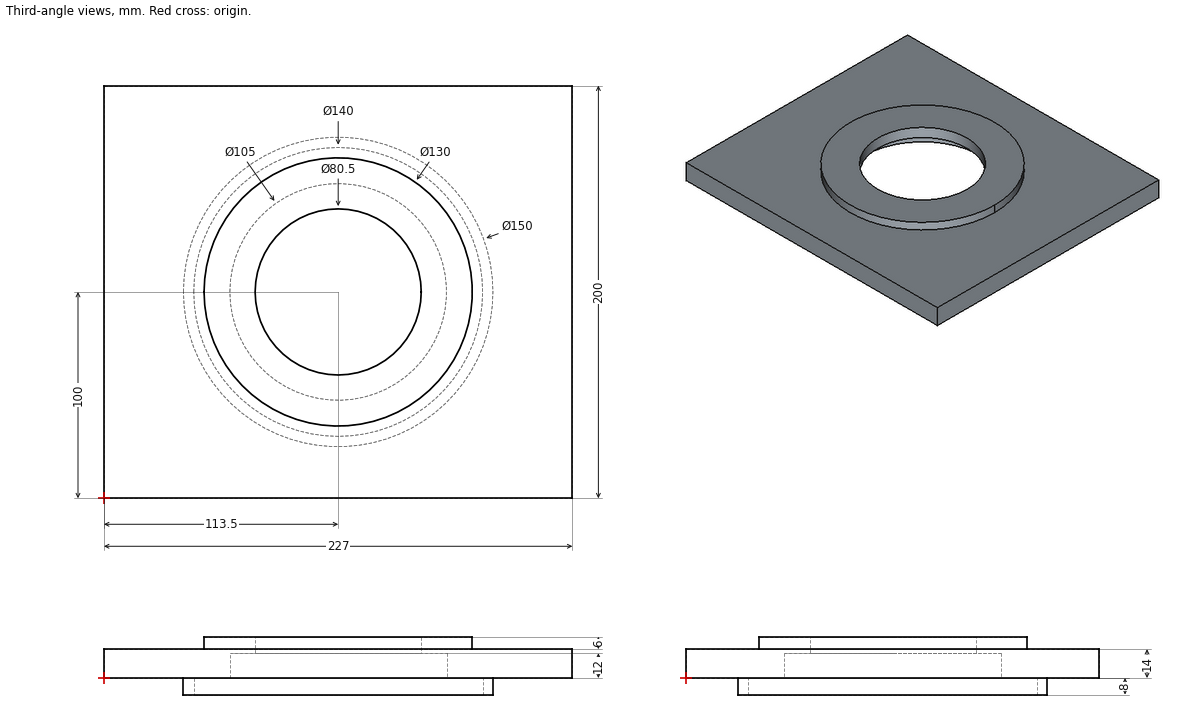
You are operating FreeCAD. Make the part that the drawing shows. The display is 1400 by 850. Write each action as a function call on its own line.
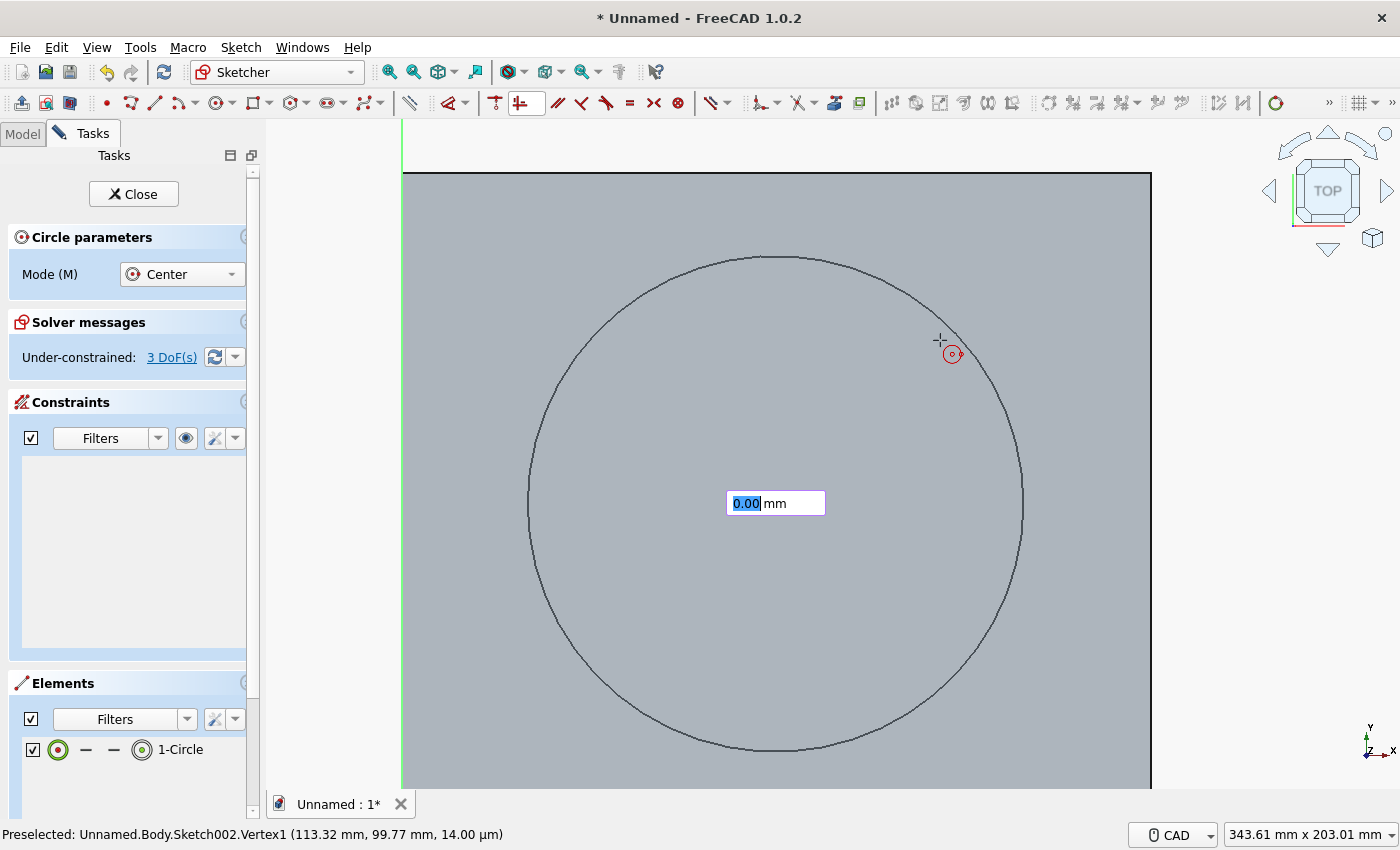
click(940, 340)
key(Escape)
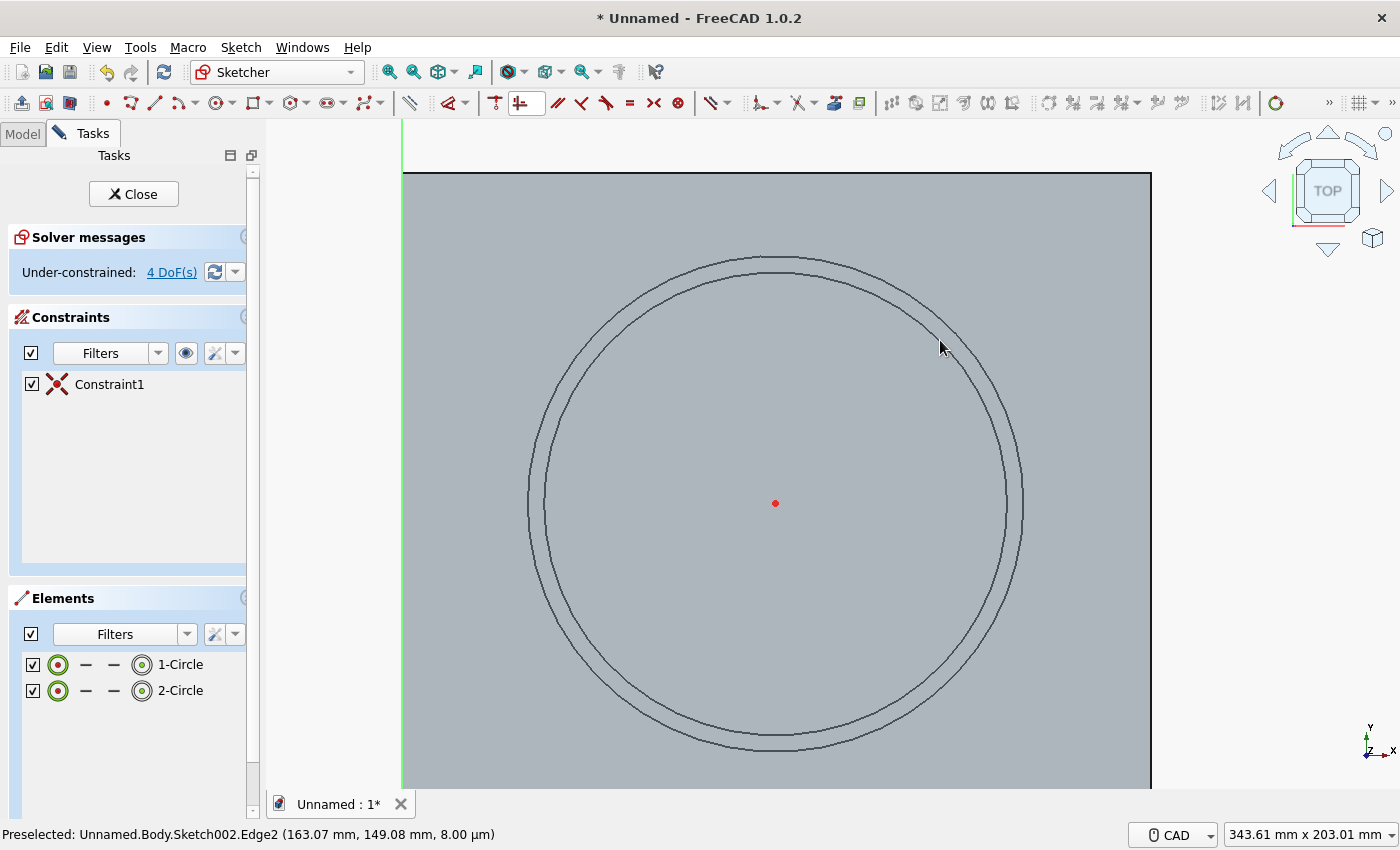
click(448, 104)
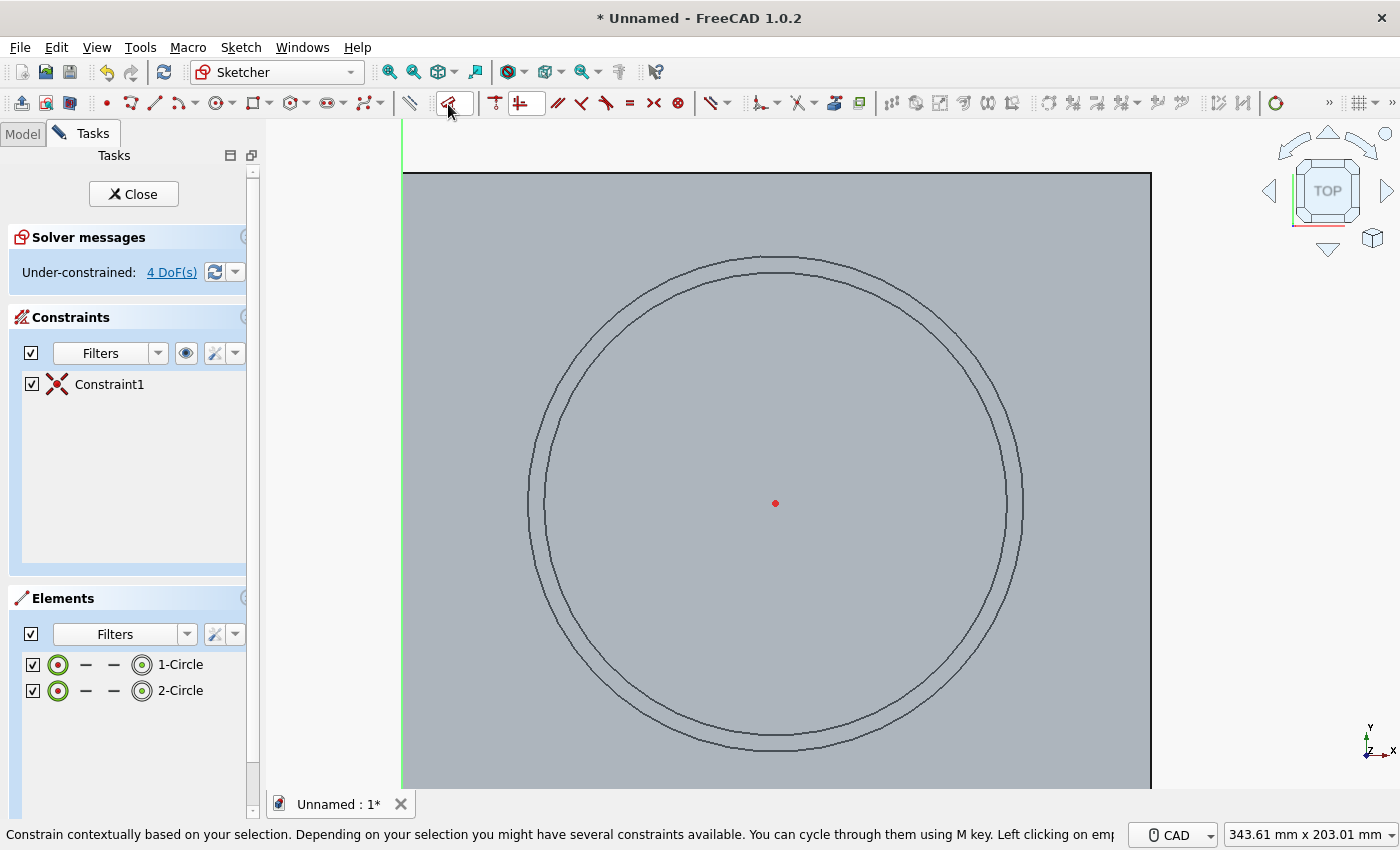
click(950, 328)
click(973, 305)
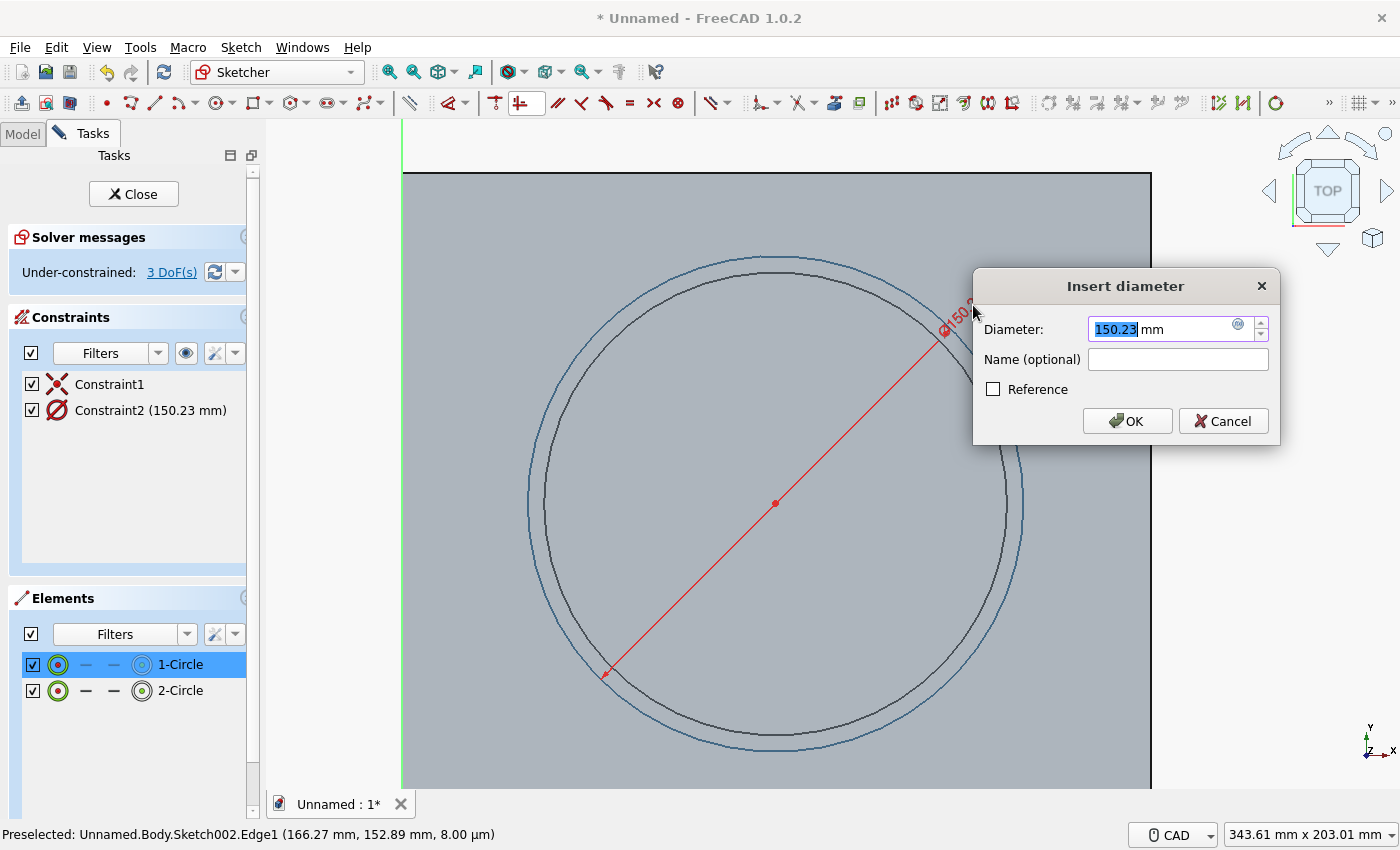
text(150)
key(Return)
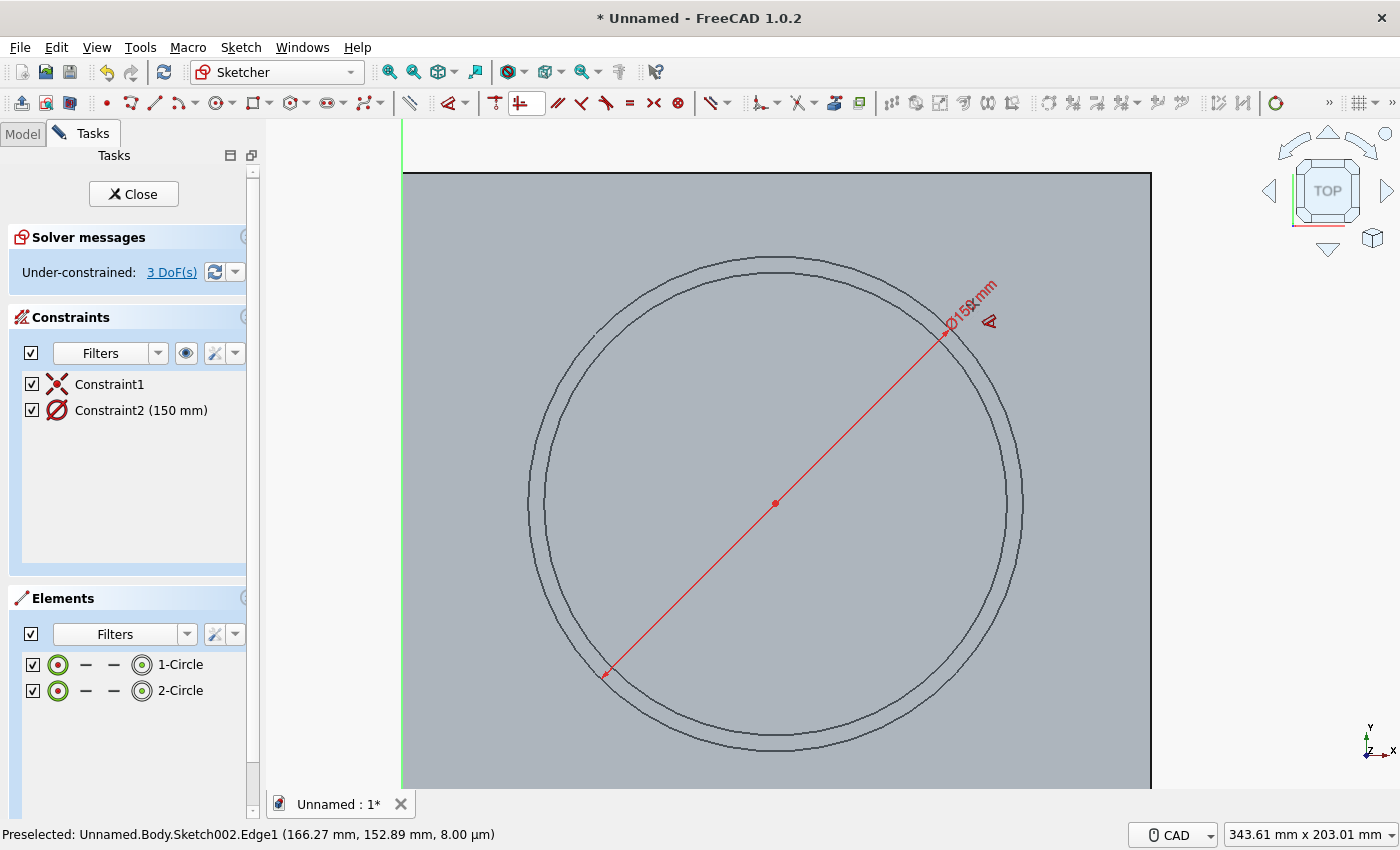
click(939, 340)
click(1028, 429)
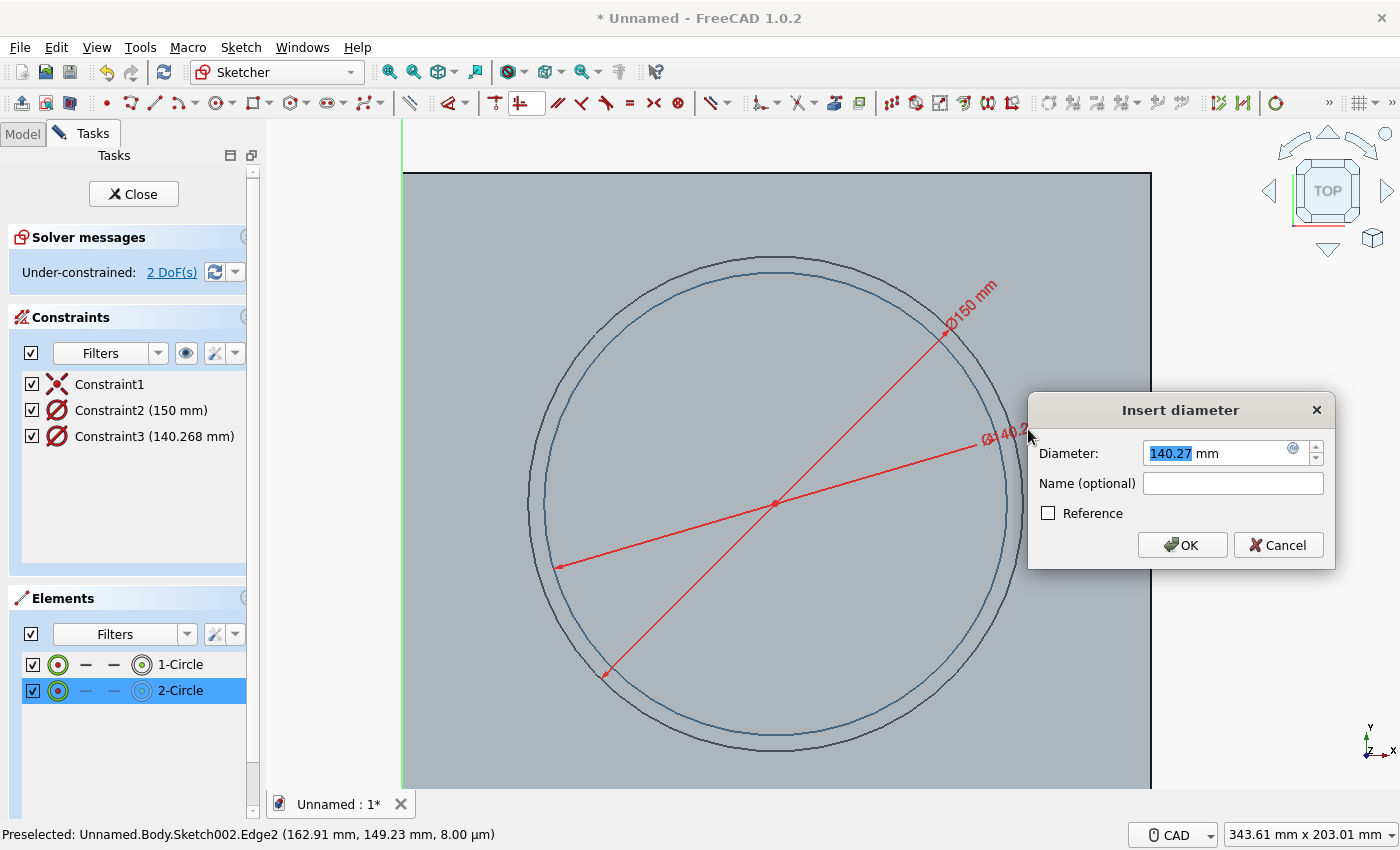
text(140)
key(Return)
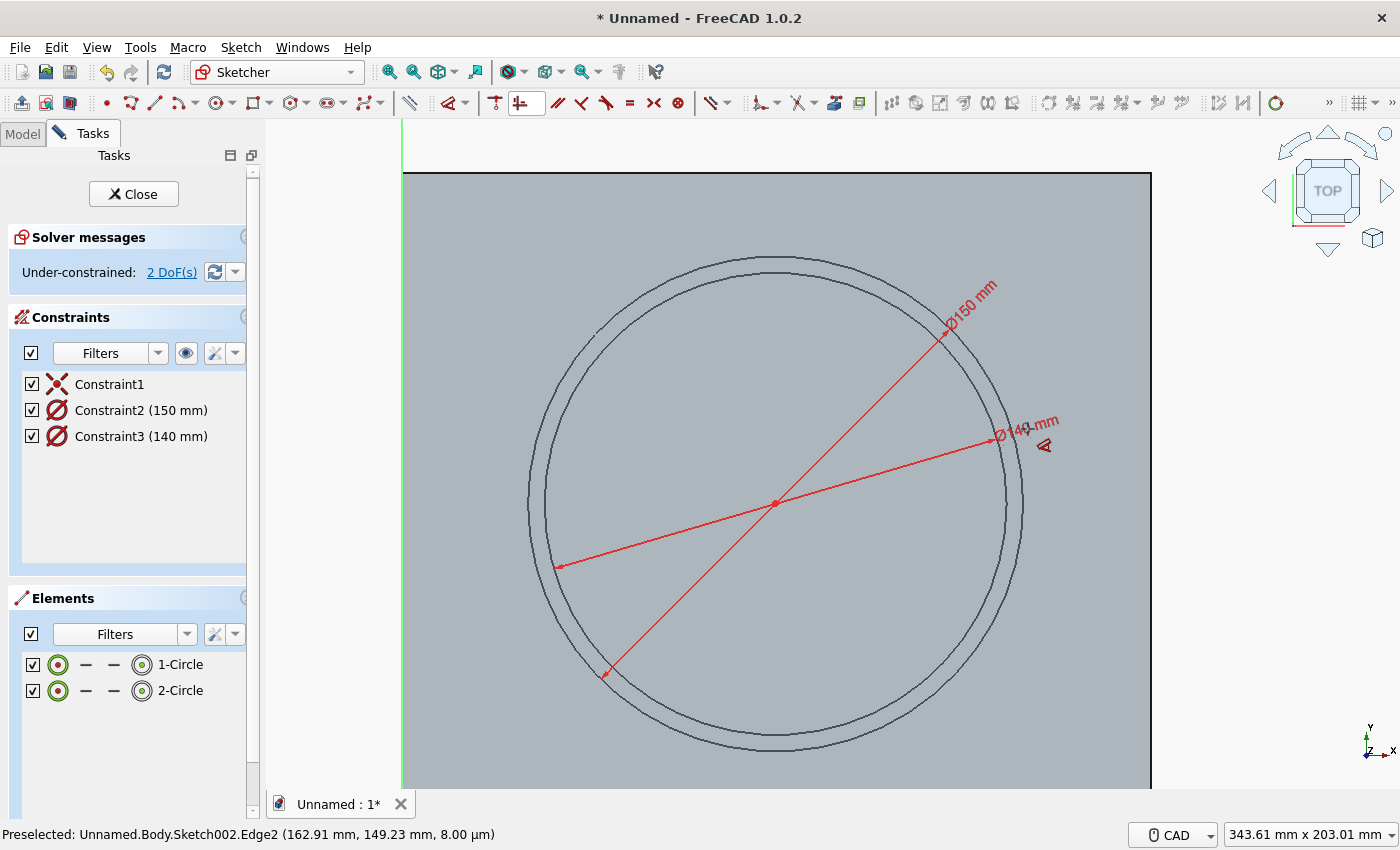
click(776, 504)
click(368, 632)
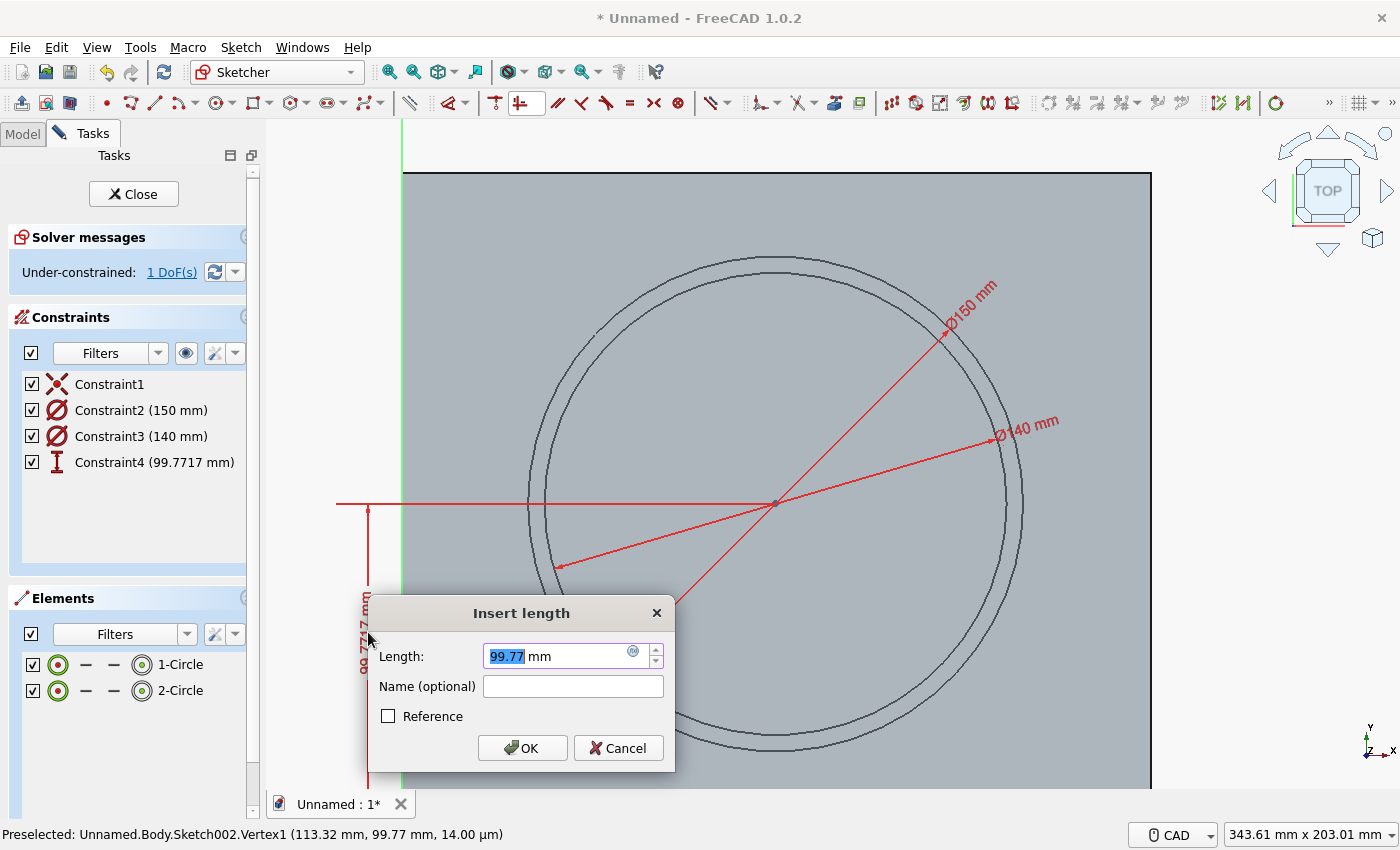
text(100)
key(Return)